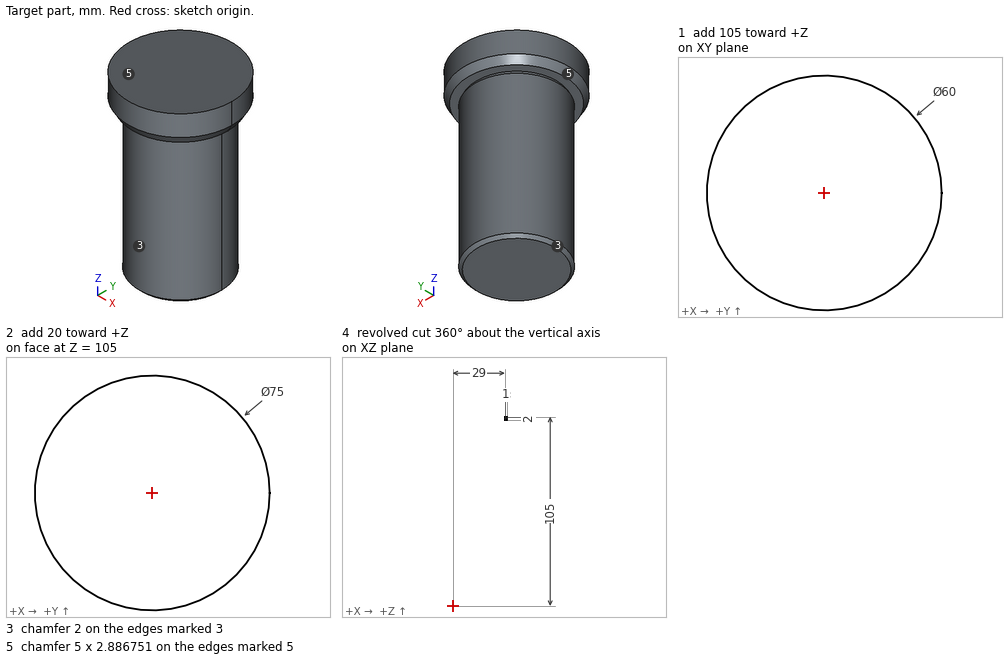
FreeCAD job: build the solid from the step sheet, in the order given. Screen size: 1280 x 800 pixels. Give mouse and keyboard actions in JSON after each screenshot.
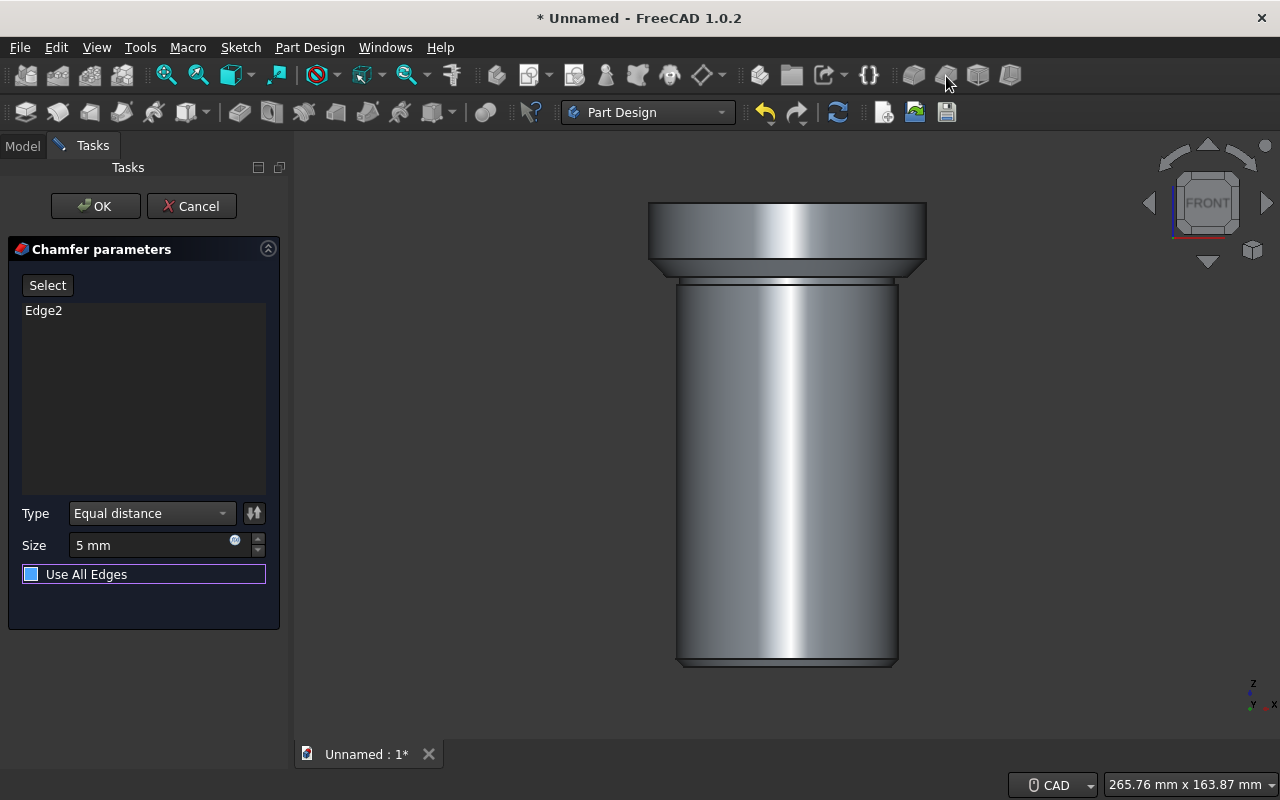
{"action": "left_click", "coordinate": [153, 514]}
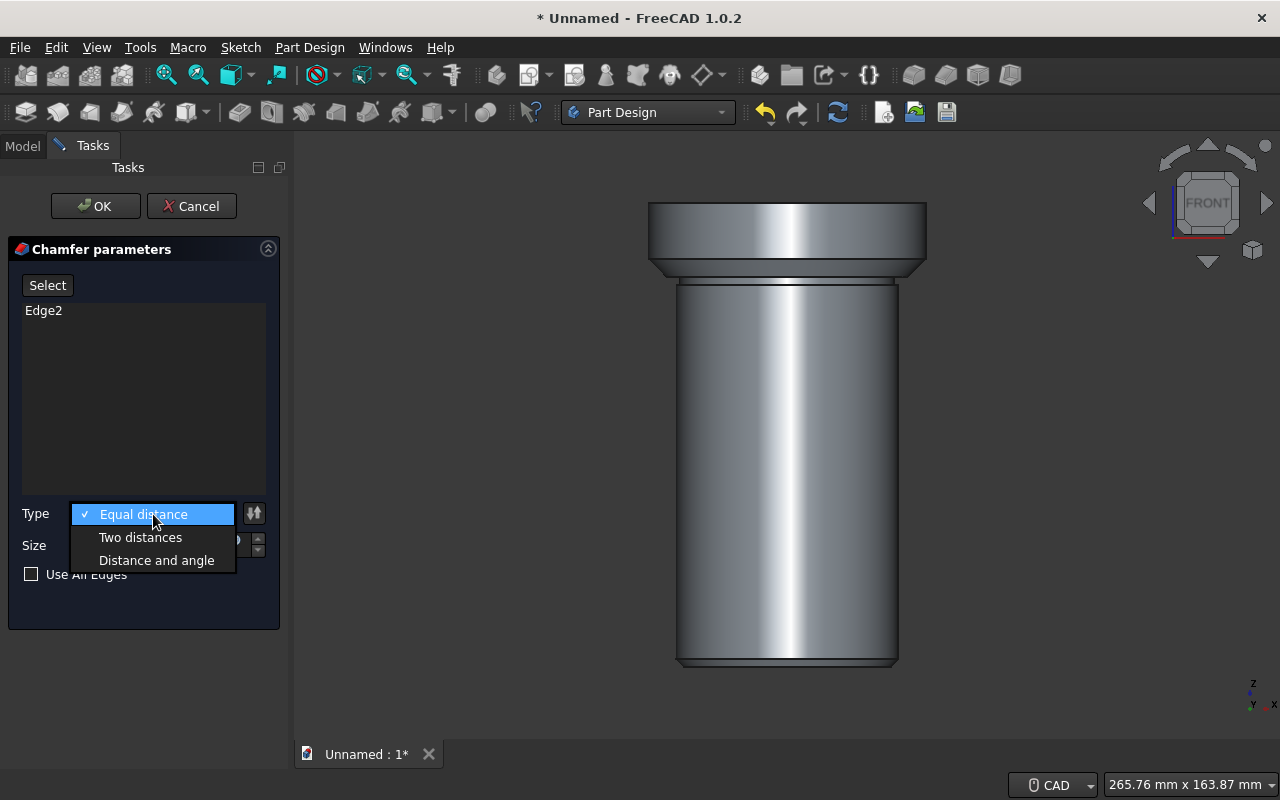
{"action": "left_click", "coordinate": [152, 538]}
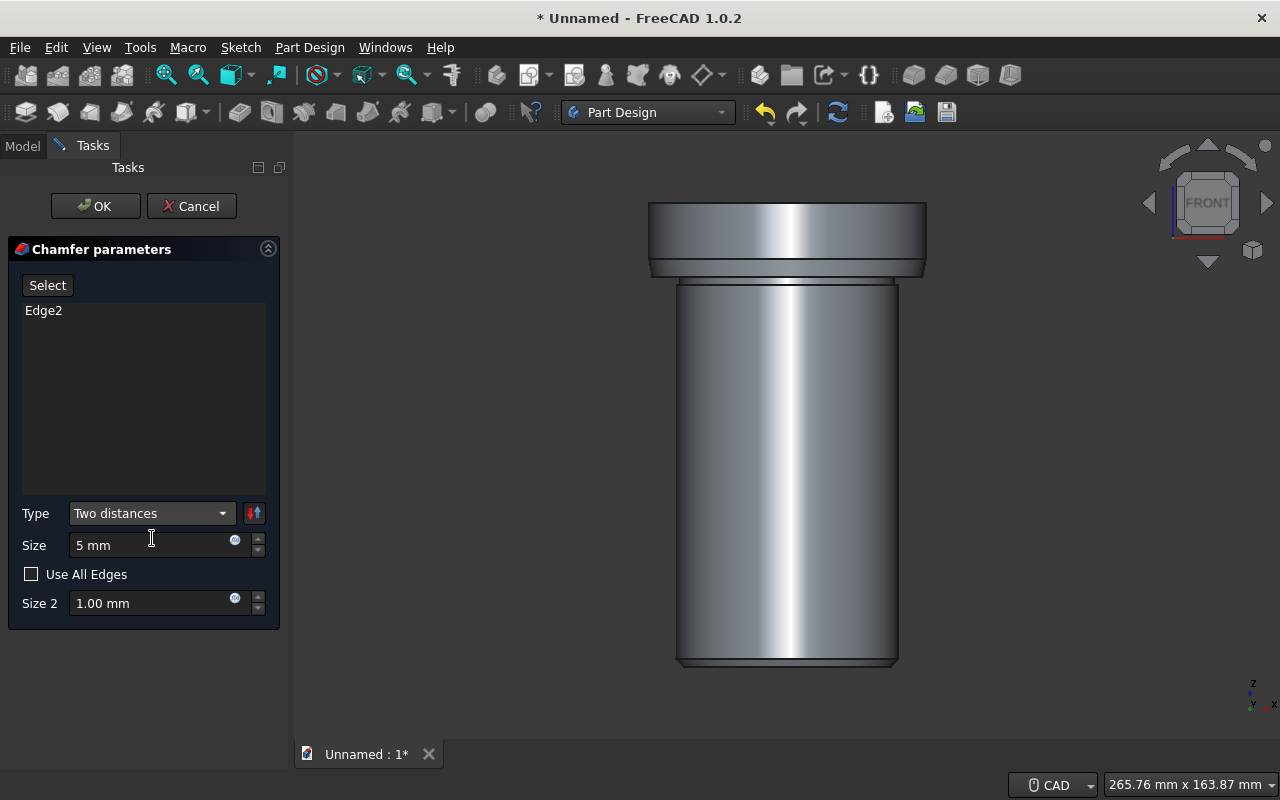
{"action": "triple_click", "coordinate": [160, 603]}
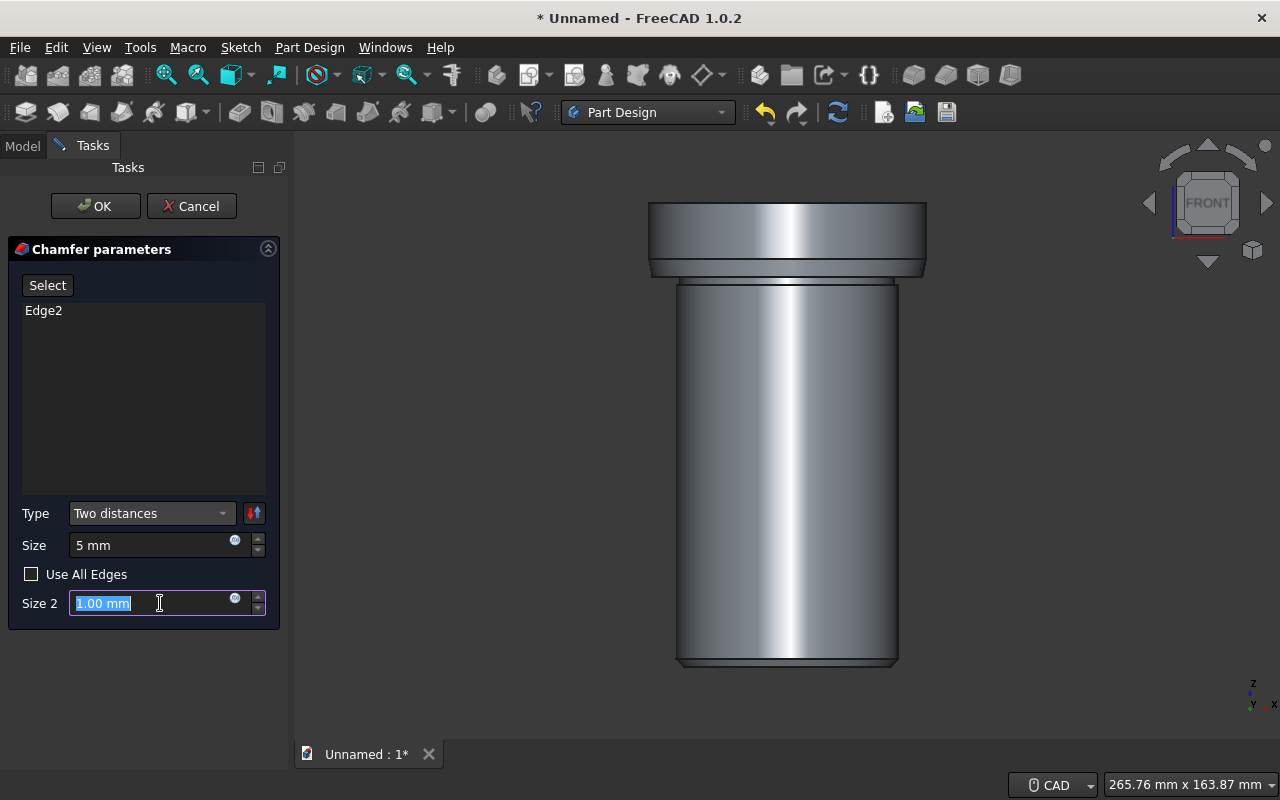
{"action": "type", "text": "2.886751"}
{"action": "key", "text": "Tab"}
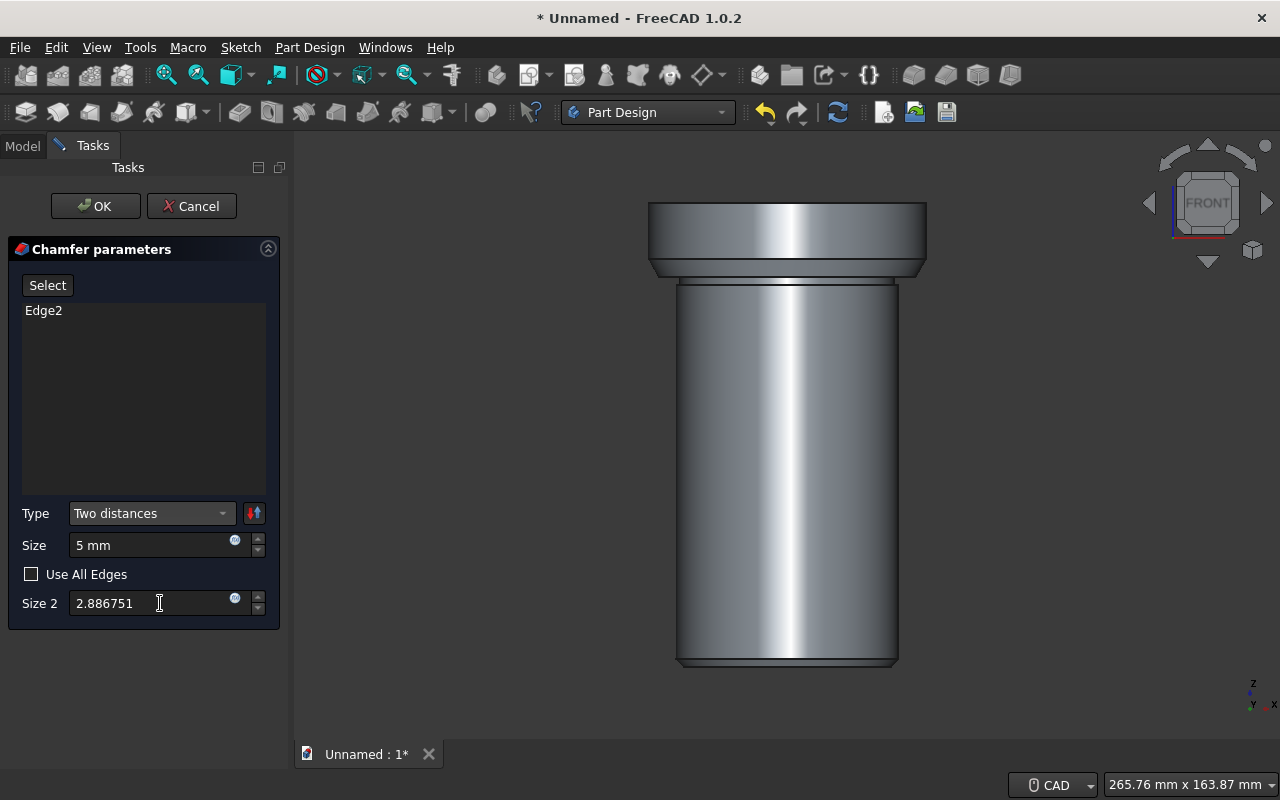
{"action": "left_click", "coordinate": [96, 206]}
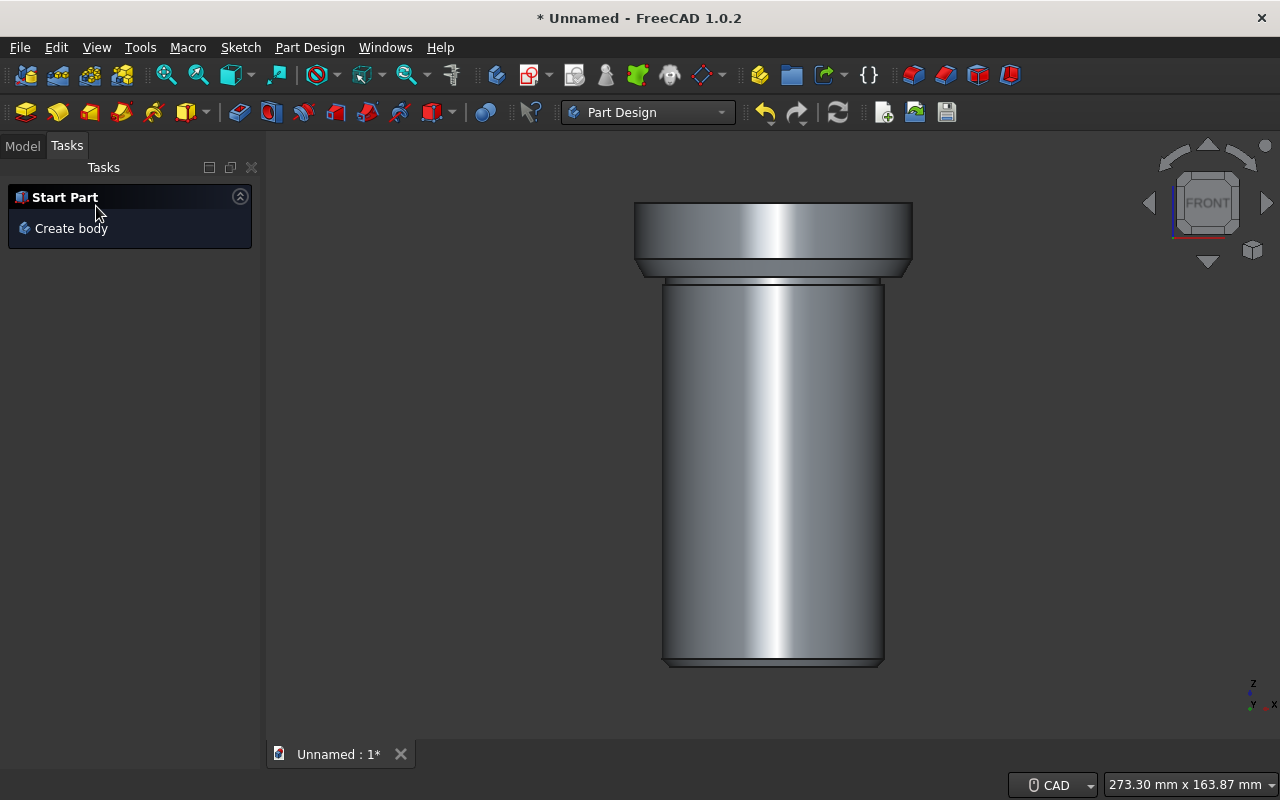
{"action": "key", "text": "0"}